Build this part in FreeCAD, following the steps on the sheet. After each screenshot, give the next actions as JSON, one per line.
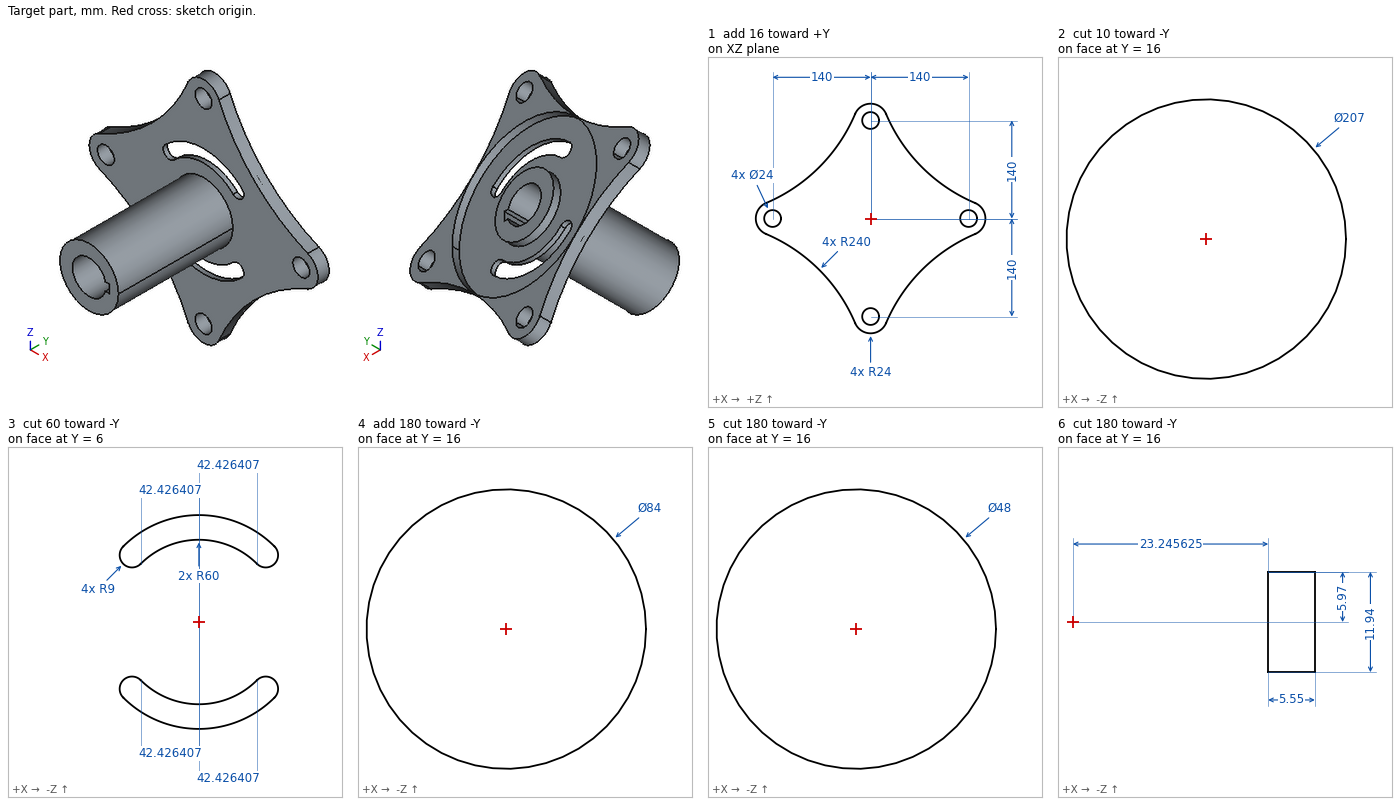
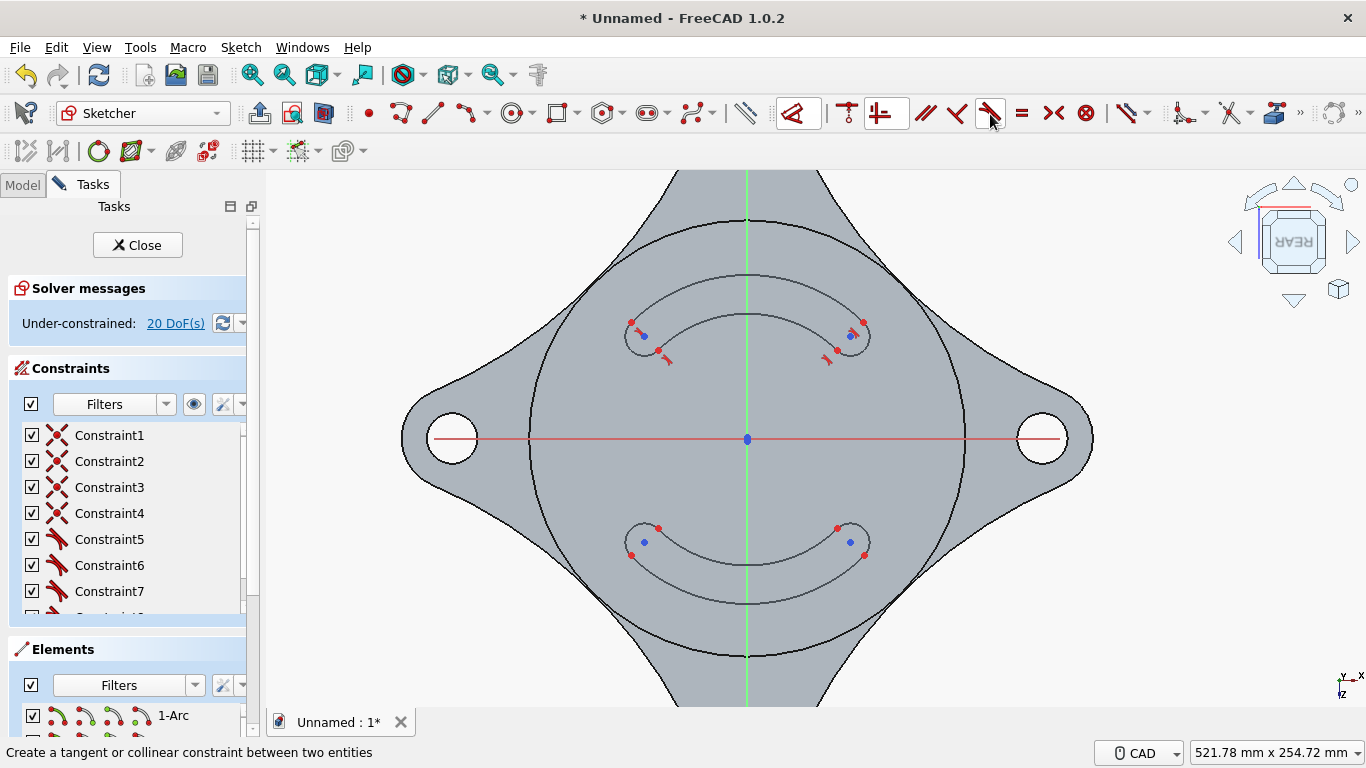
{"action": "left_click", "coordinate": [708, 559]}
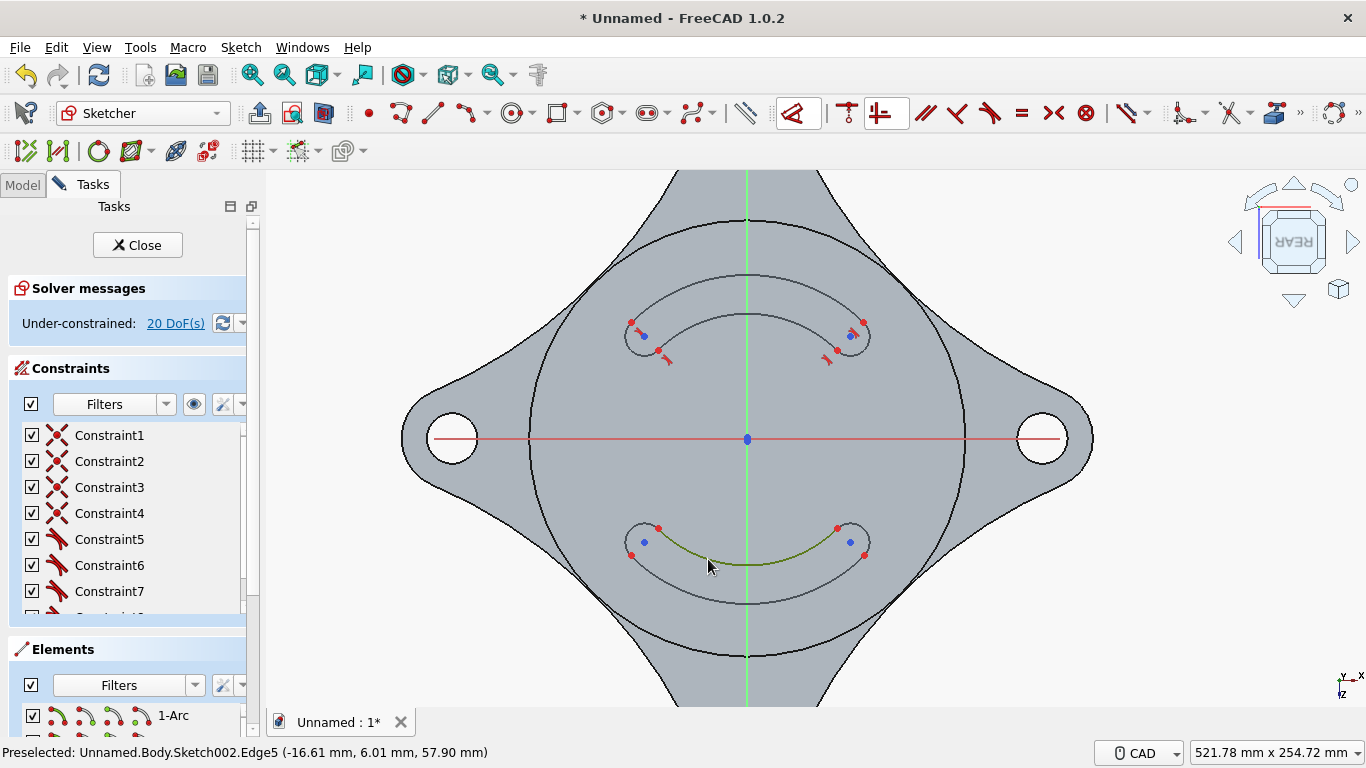
{"action": "left_click", "coordinate": [642, 524]}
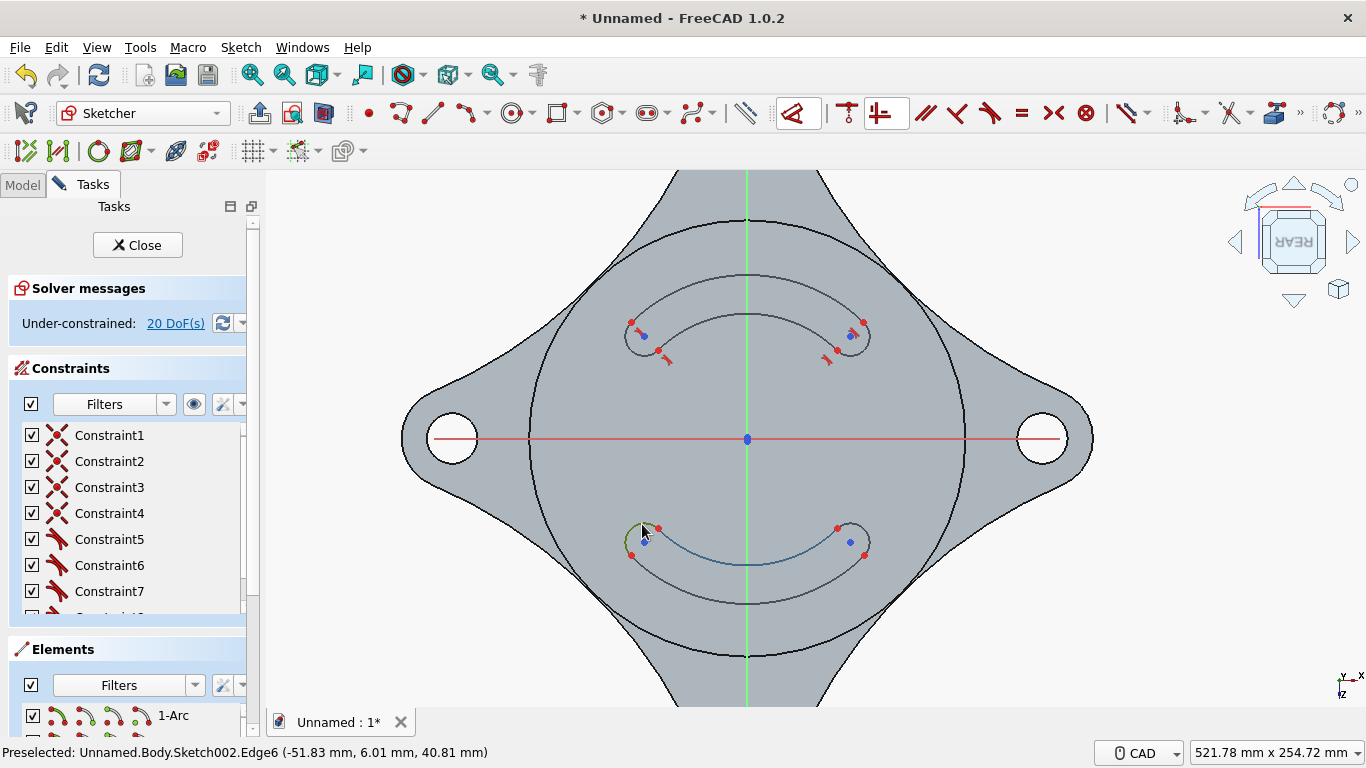
{"action": "left_click", "coordinate": [990, 114]}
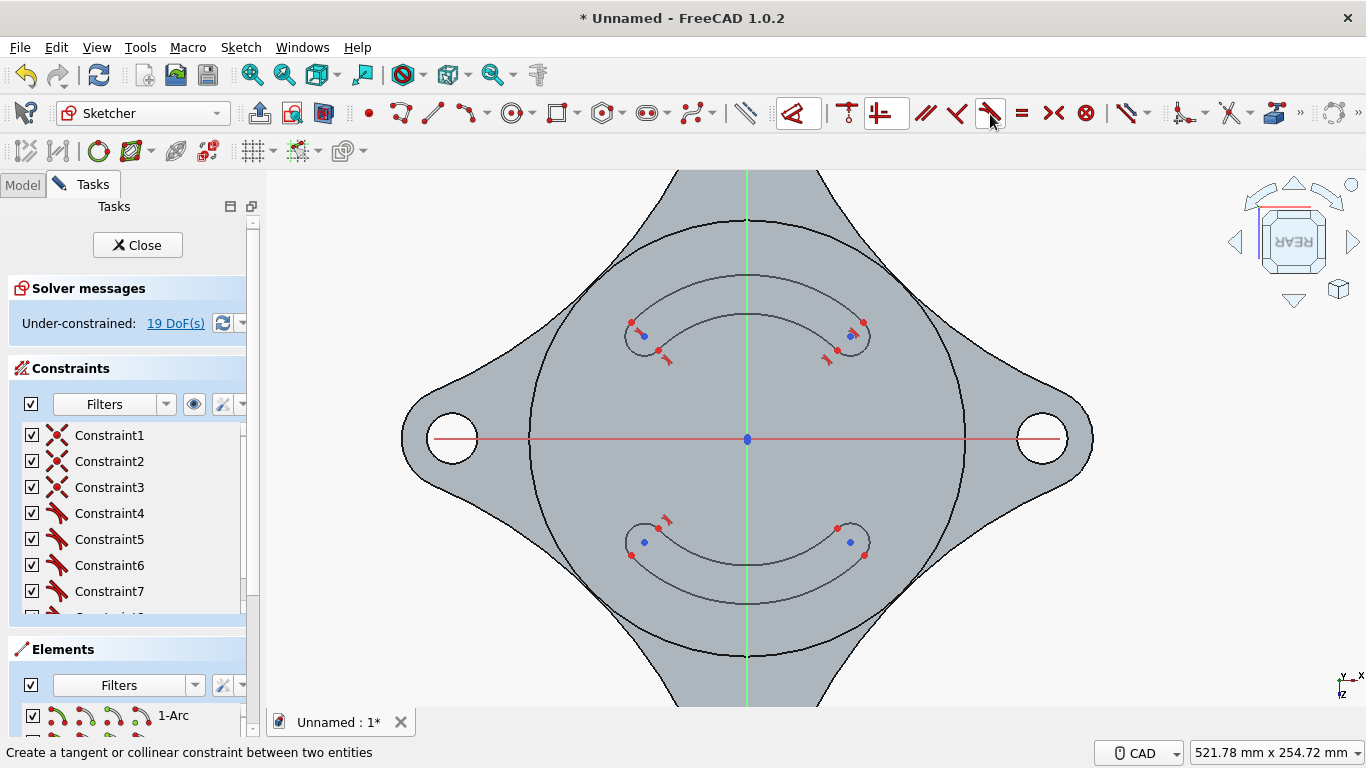
{"action": "left_click", "coordinate": [708, 559]}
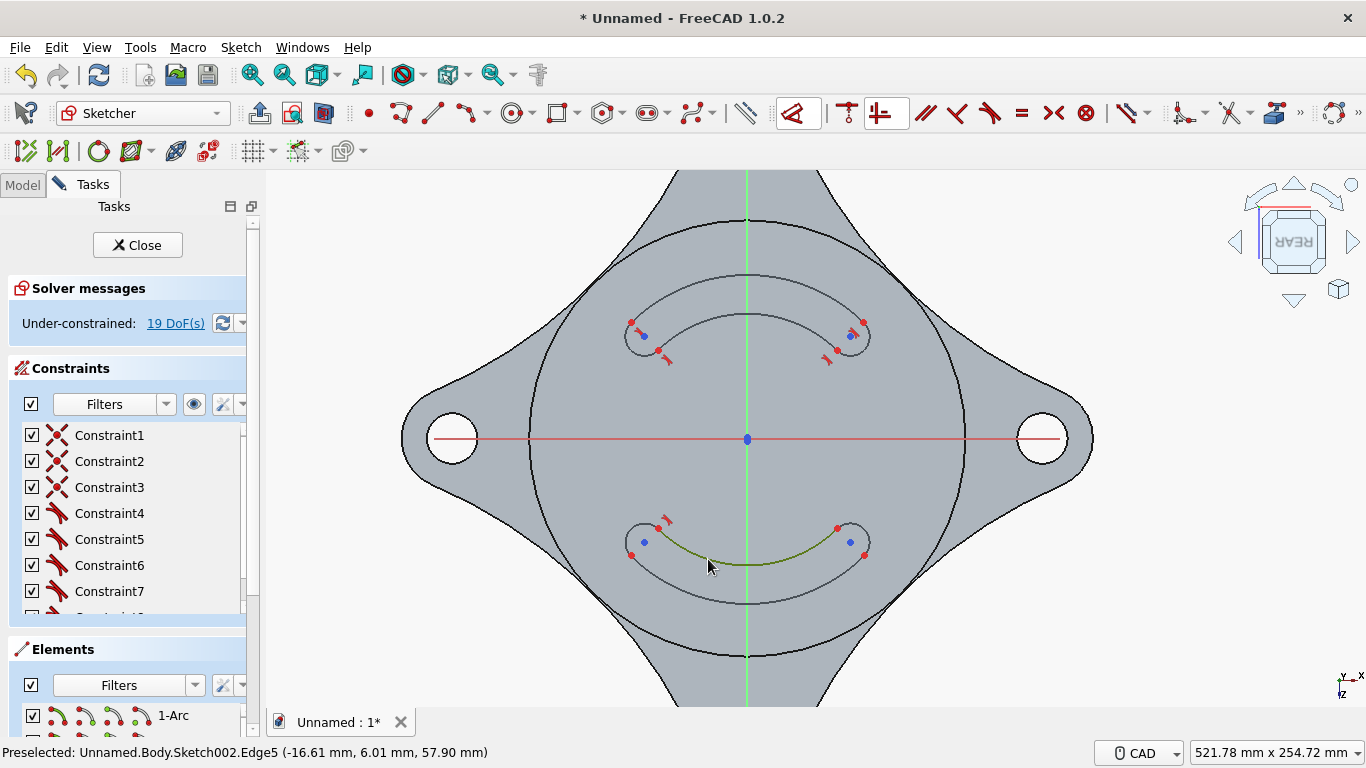
{"action": "left_click", "coordinate": [869, 540]}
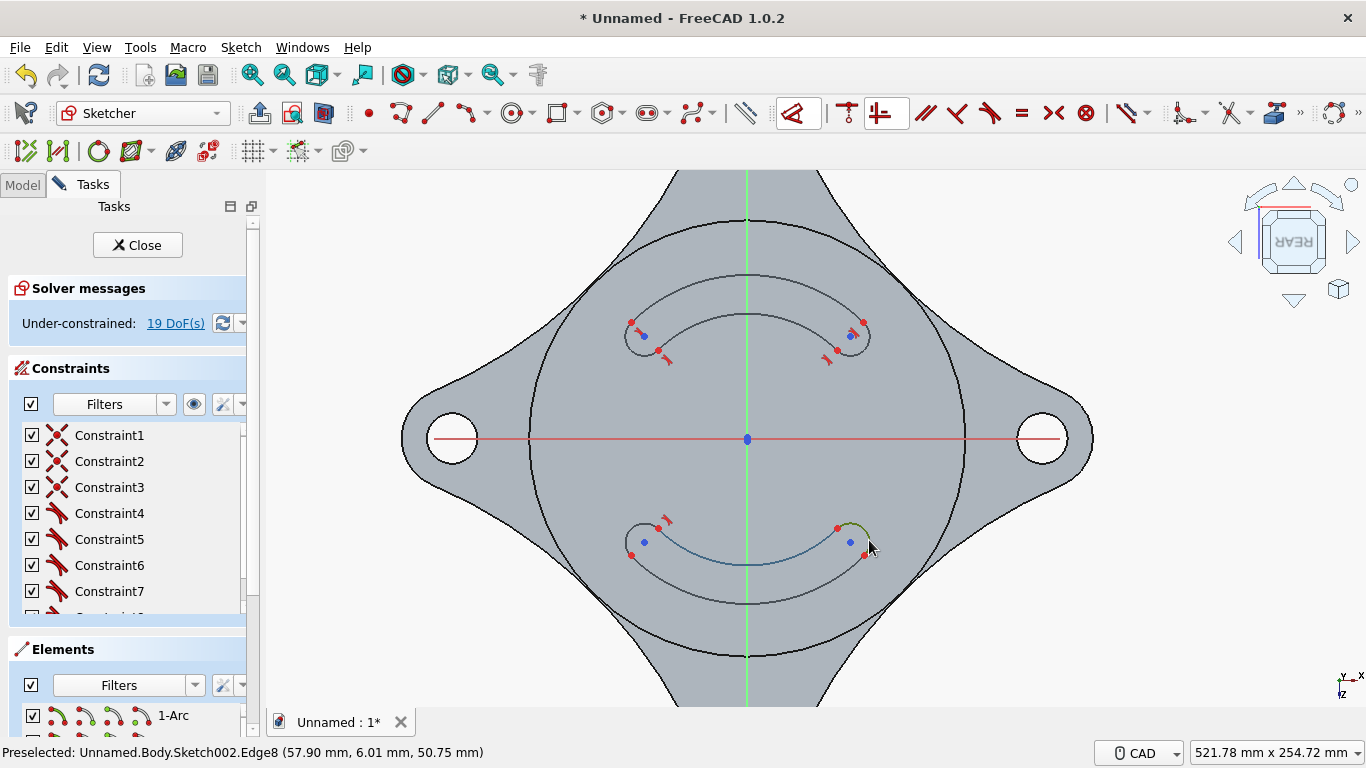
{"action": "left_click", "coordinate": [990, 114]}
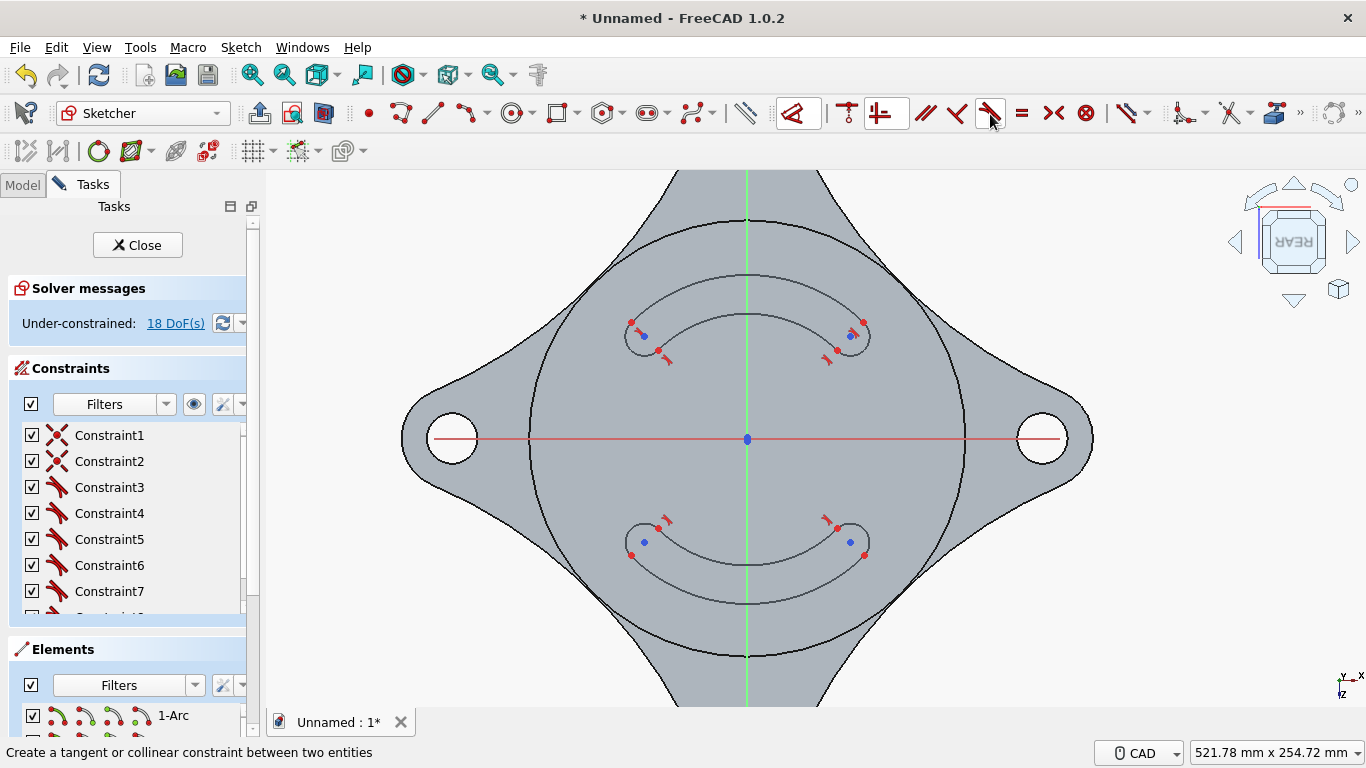
{"action": "left_click", "coordinate": [642, 524]}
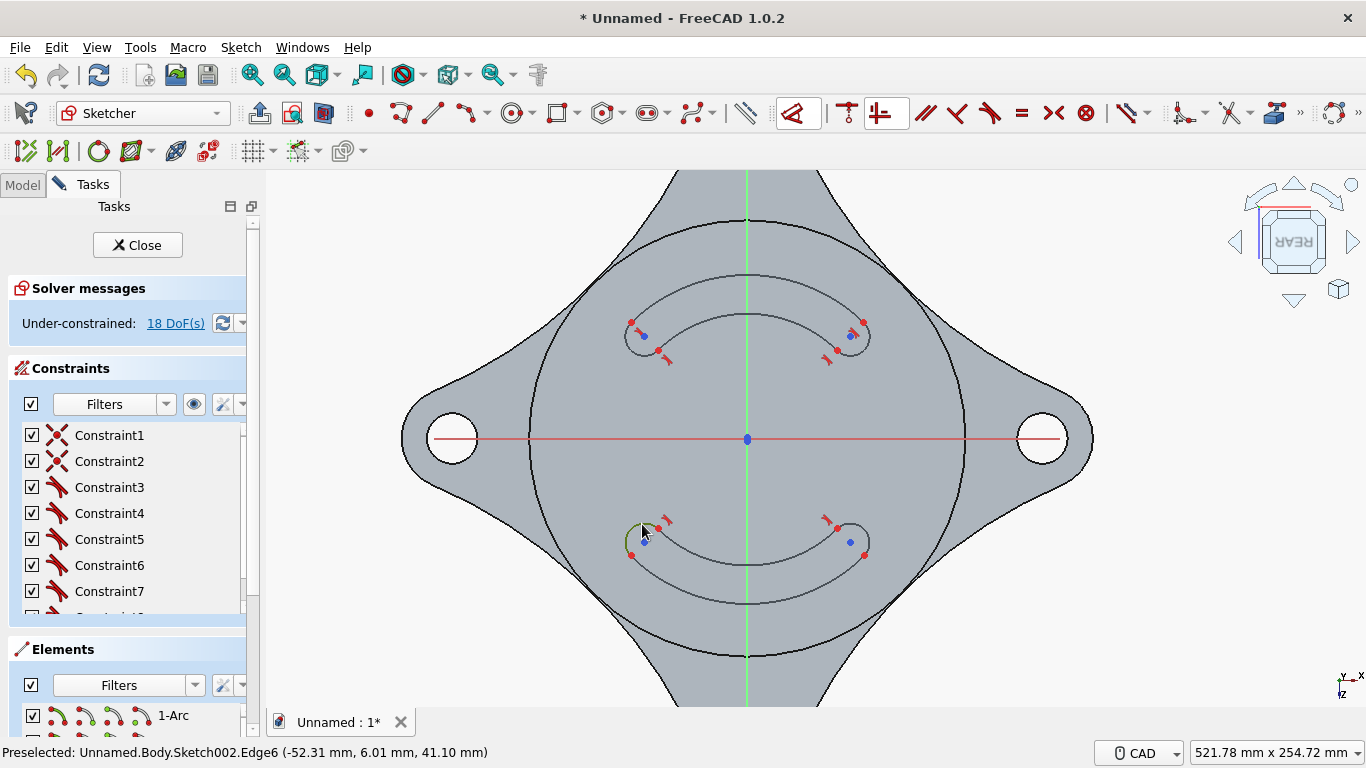
{"action": "left_click", "coordinate": [697, 596]}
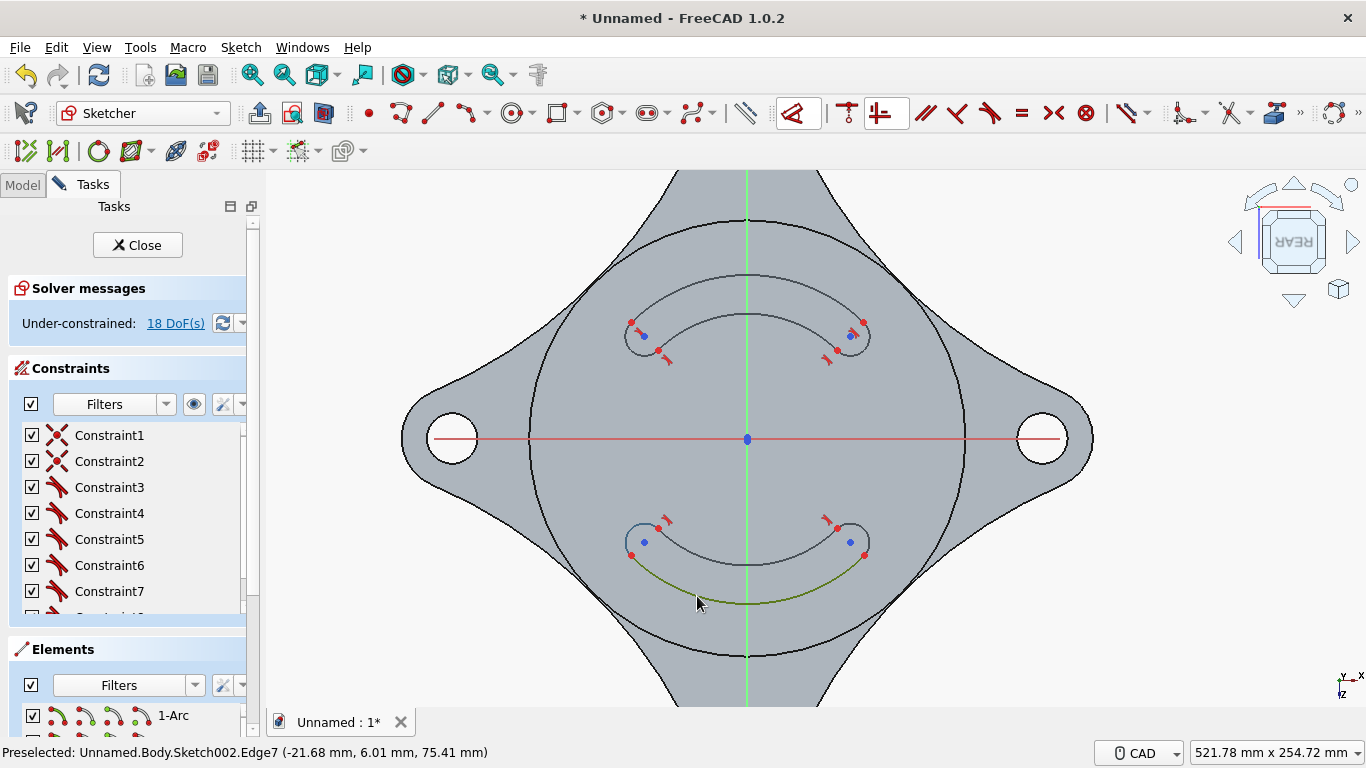
{"action": "left_click", "coordinate": [990, 114]}